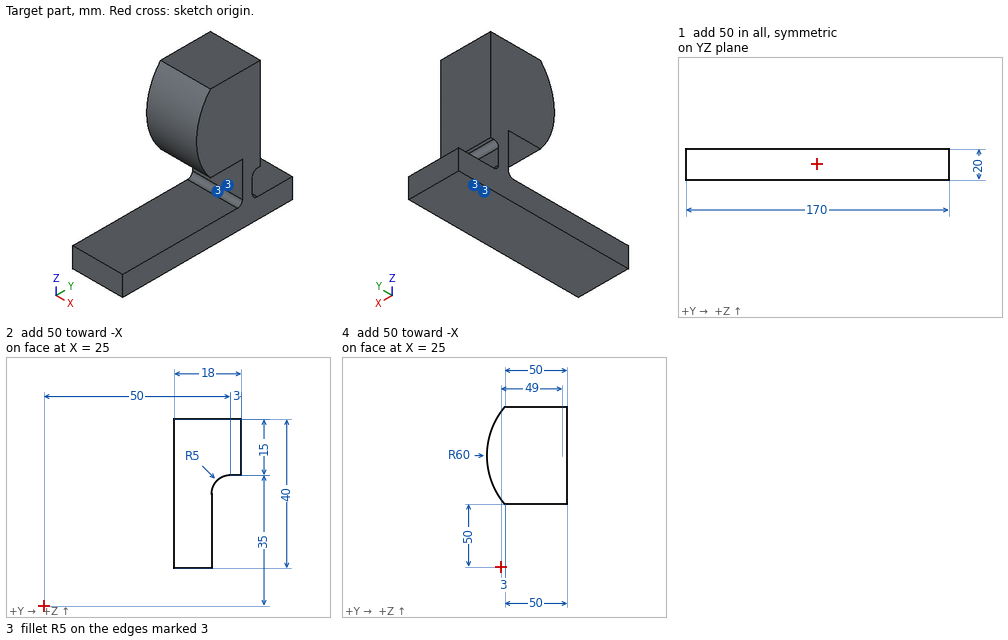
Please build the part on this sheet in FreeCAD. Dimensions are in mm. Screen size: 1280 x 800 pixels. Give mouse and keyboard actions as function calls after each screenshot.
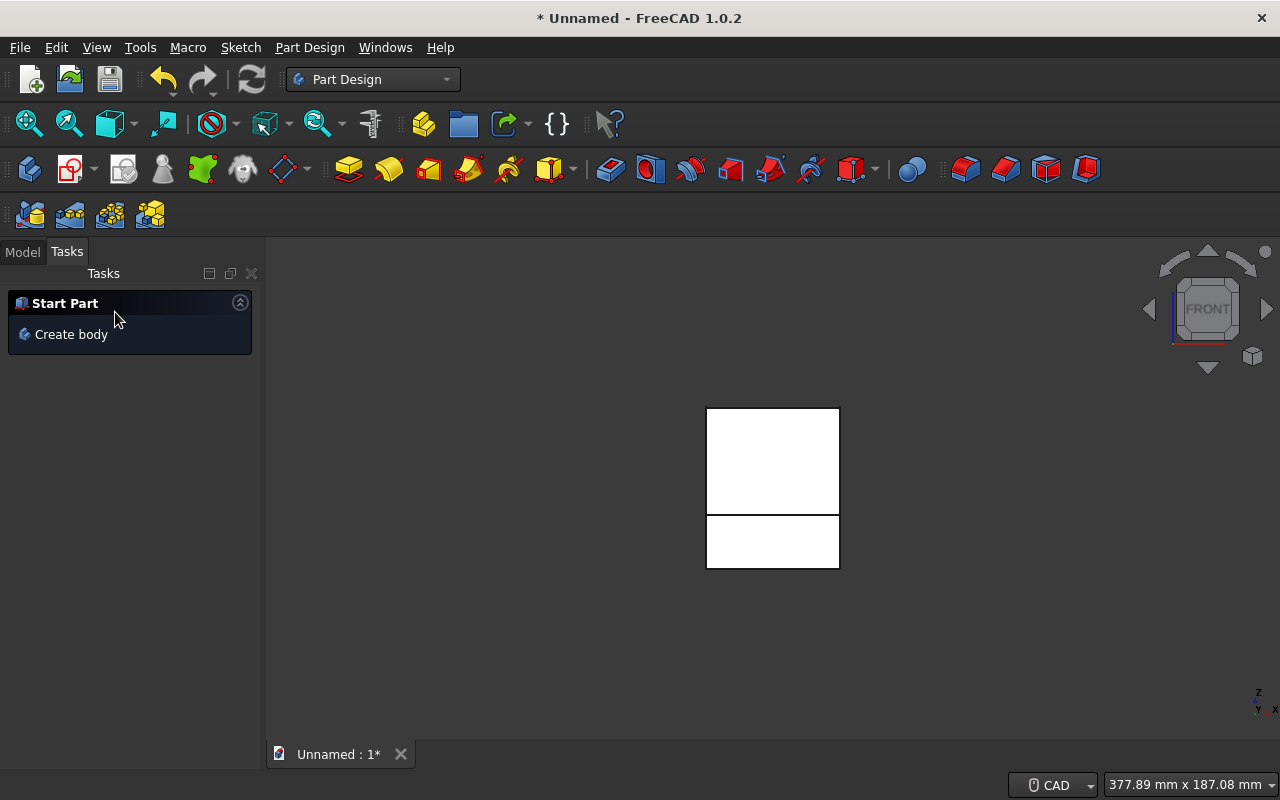
key(3)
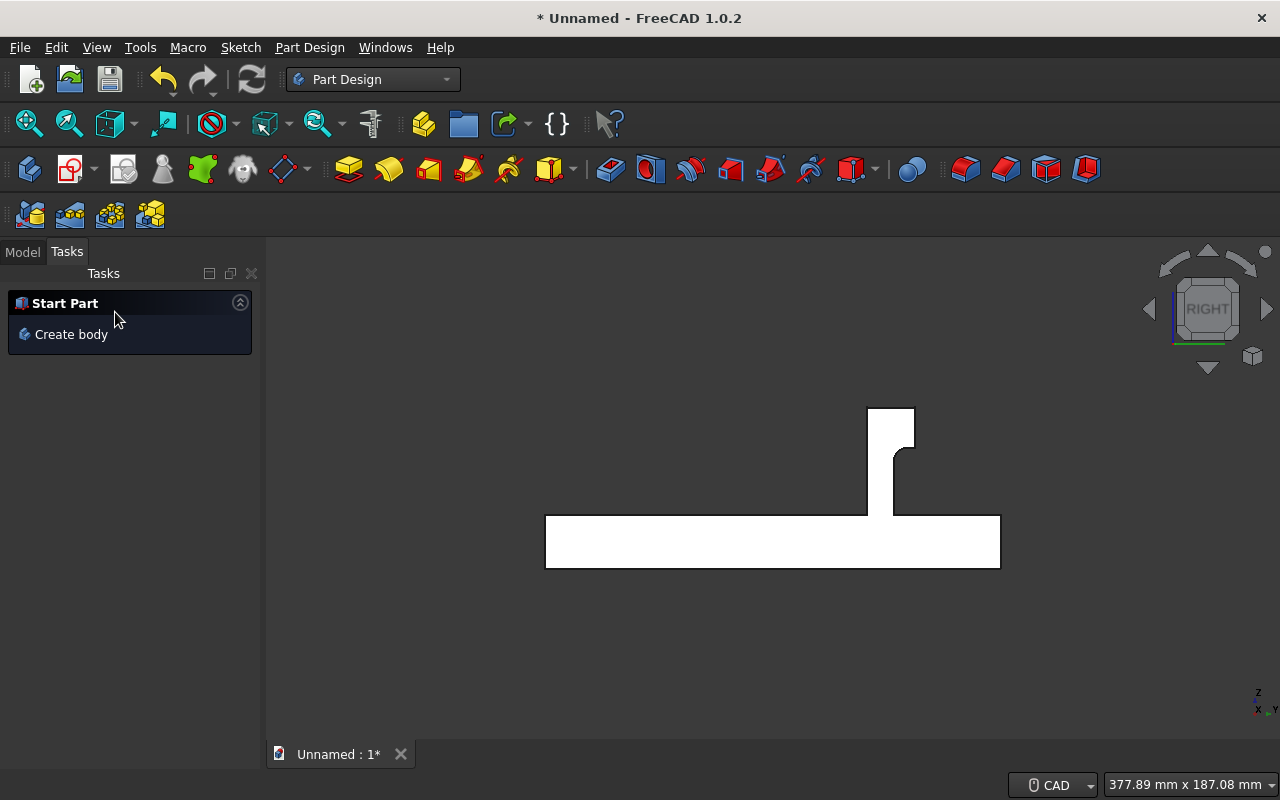
key(v)
key(f)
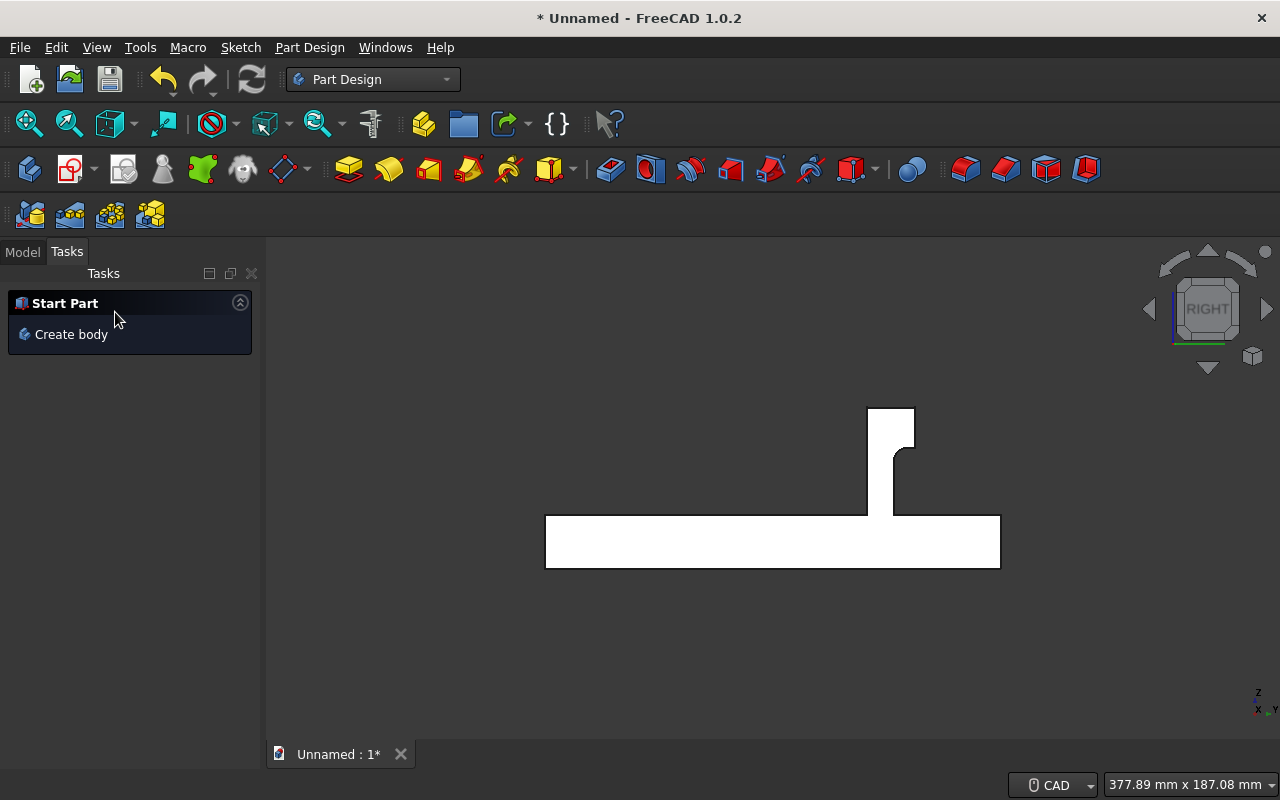
key(5)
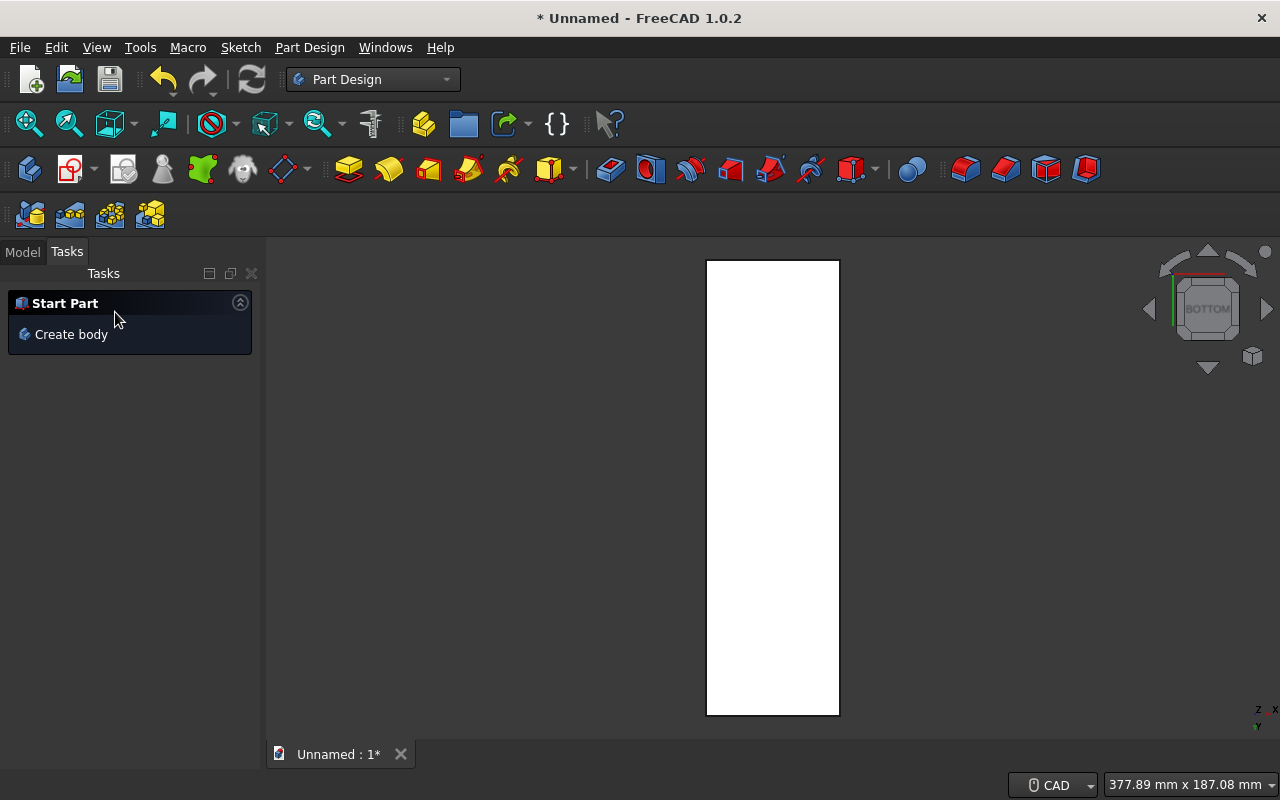
key(4)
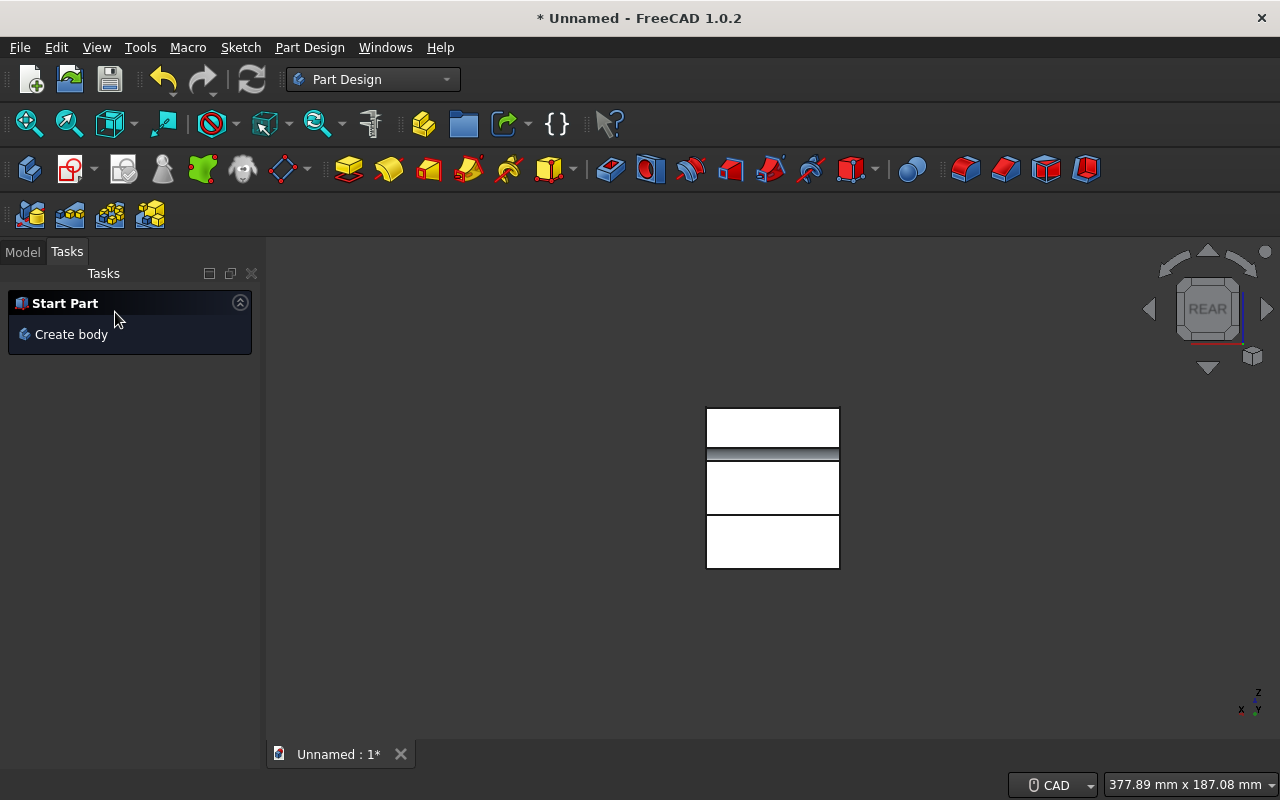
click(30, 124)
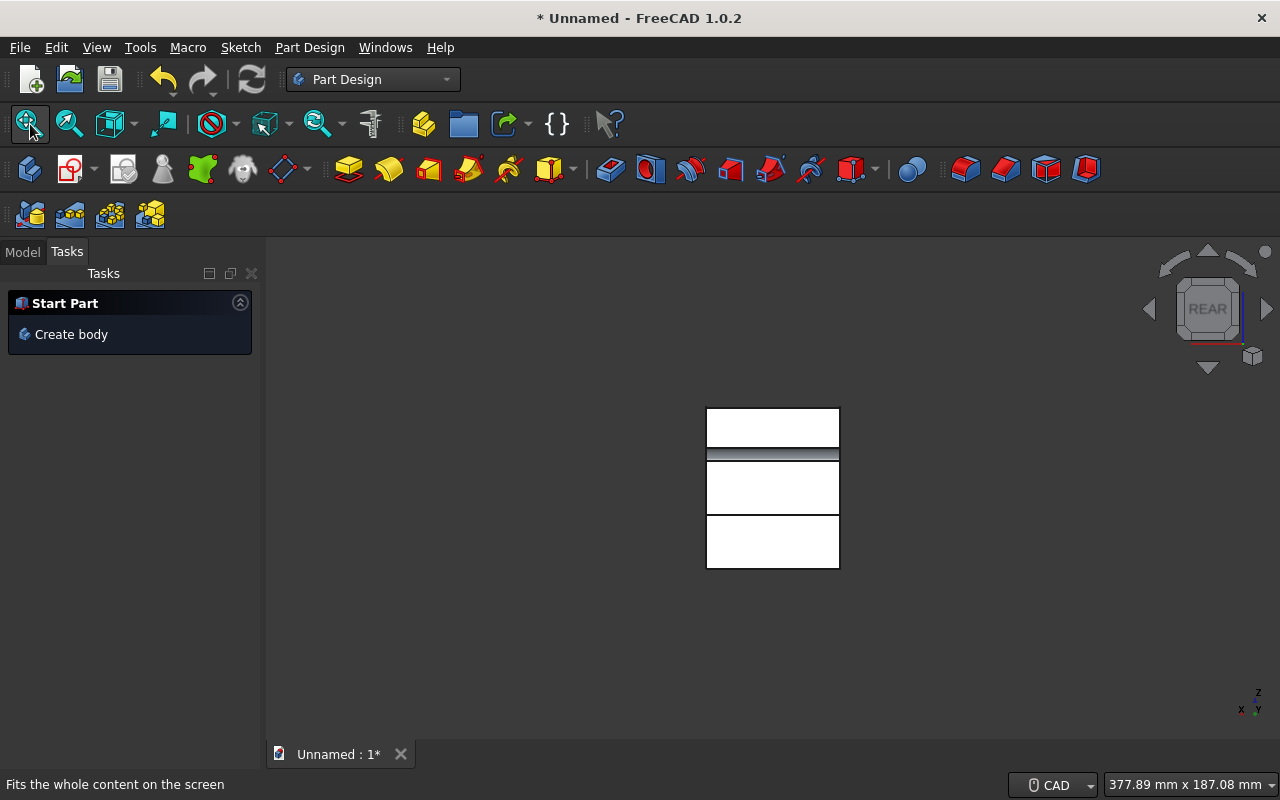
key(6)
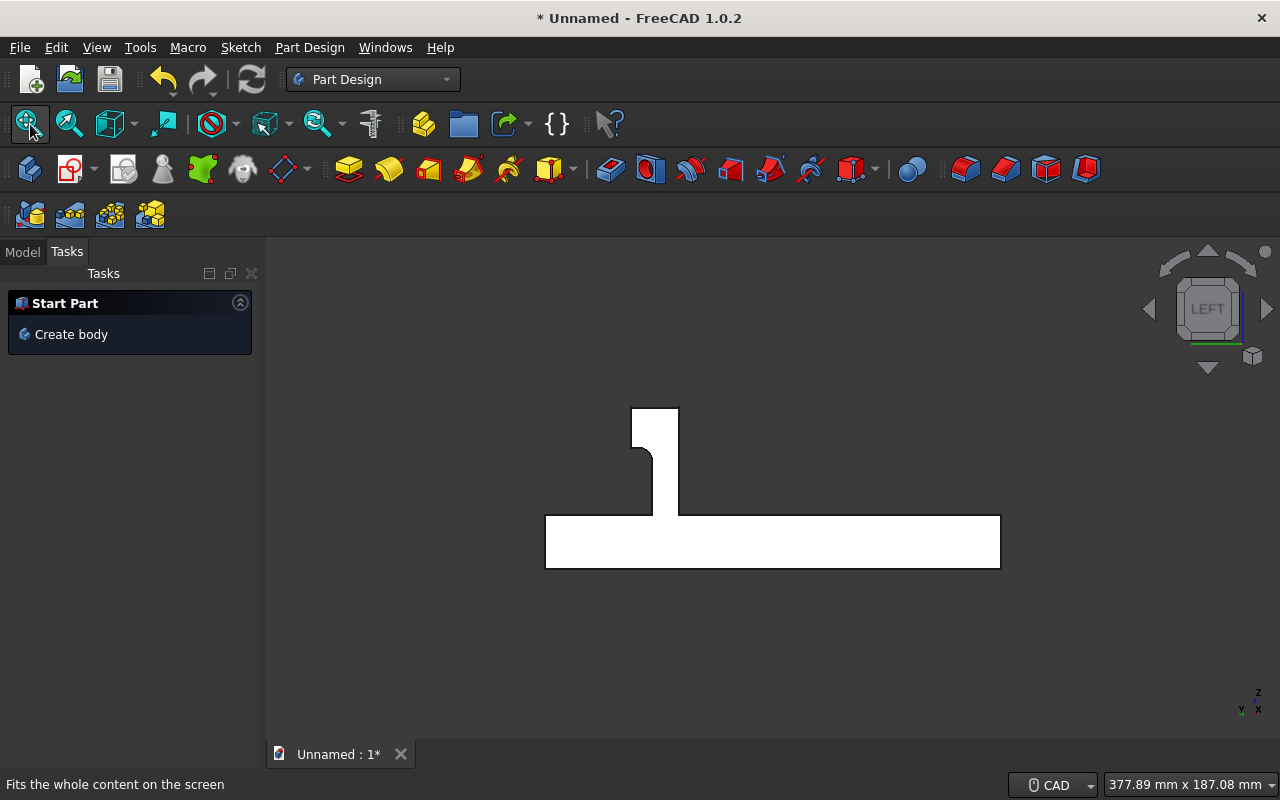
key(v)
key(f)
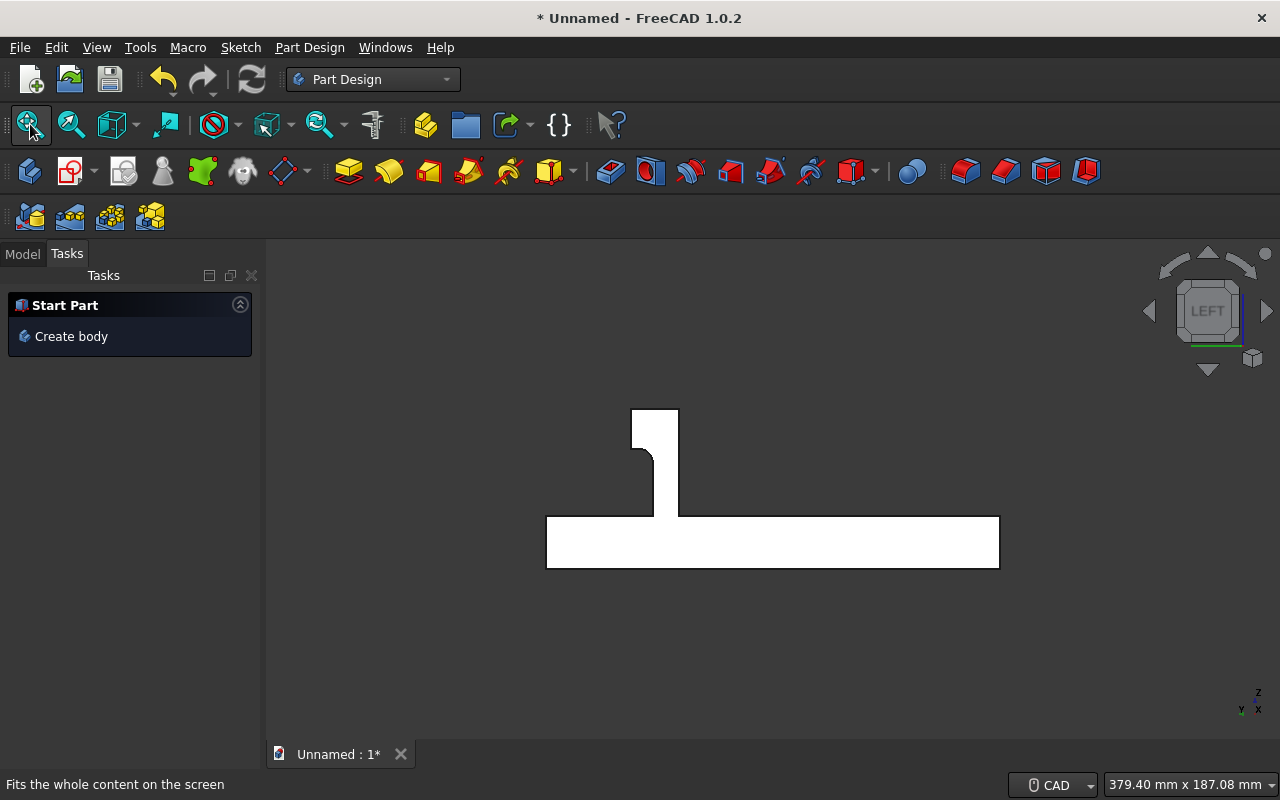
key(v)
key(3)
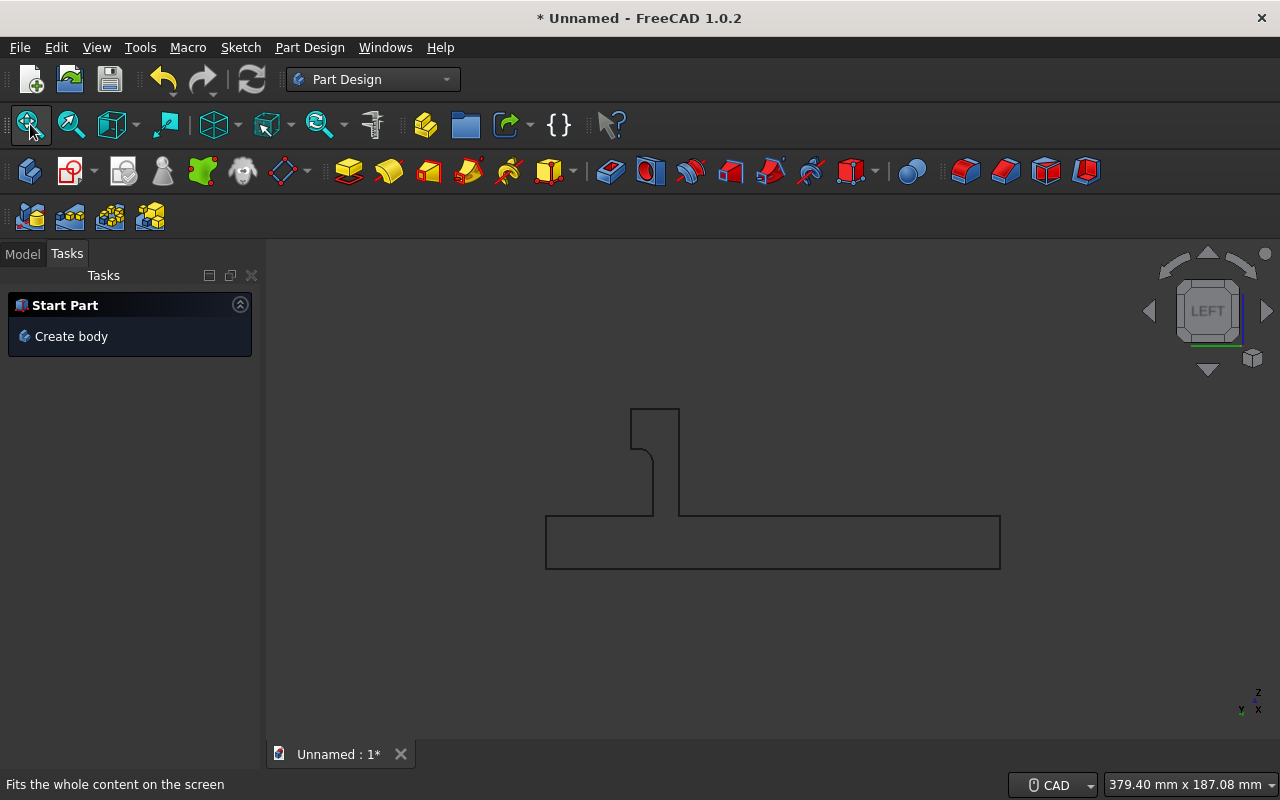
key(0)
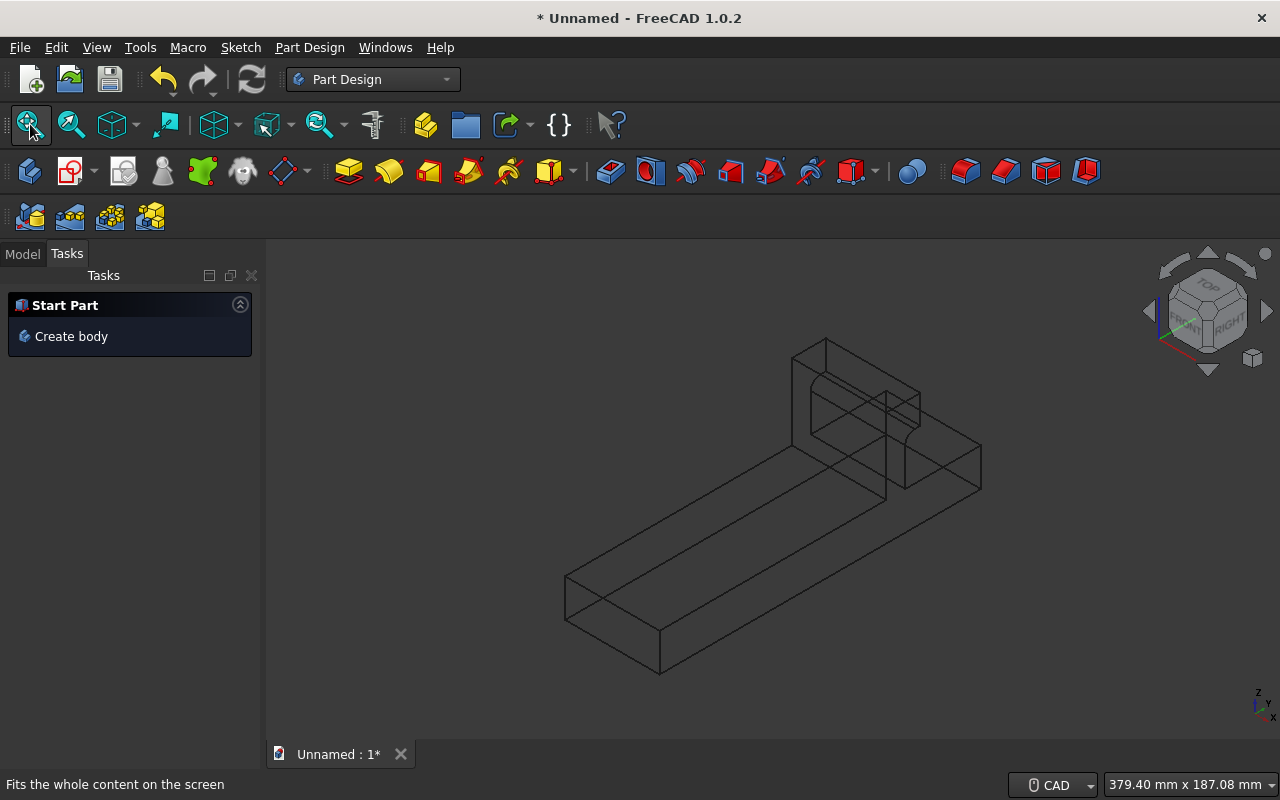
click(858, 461)